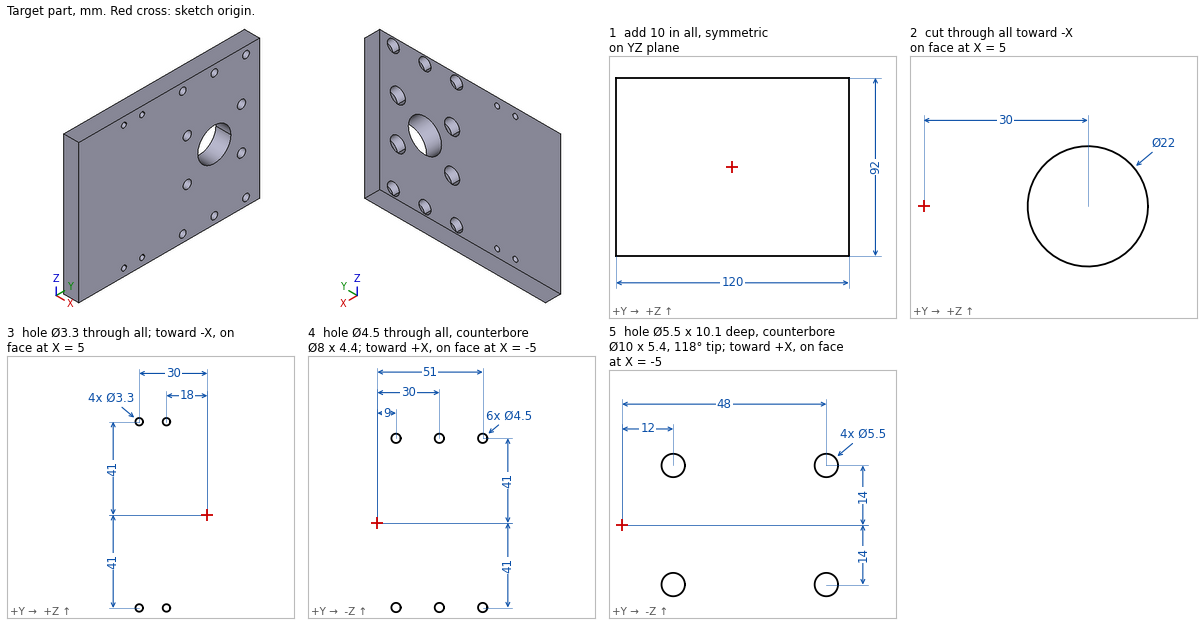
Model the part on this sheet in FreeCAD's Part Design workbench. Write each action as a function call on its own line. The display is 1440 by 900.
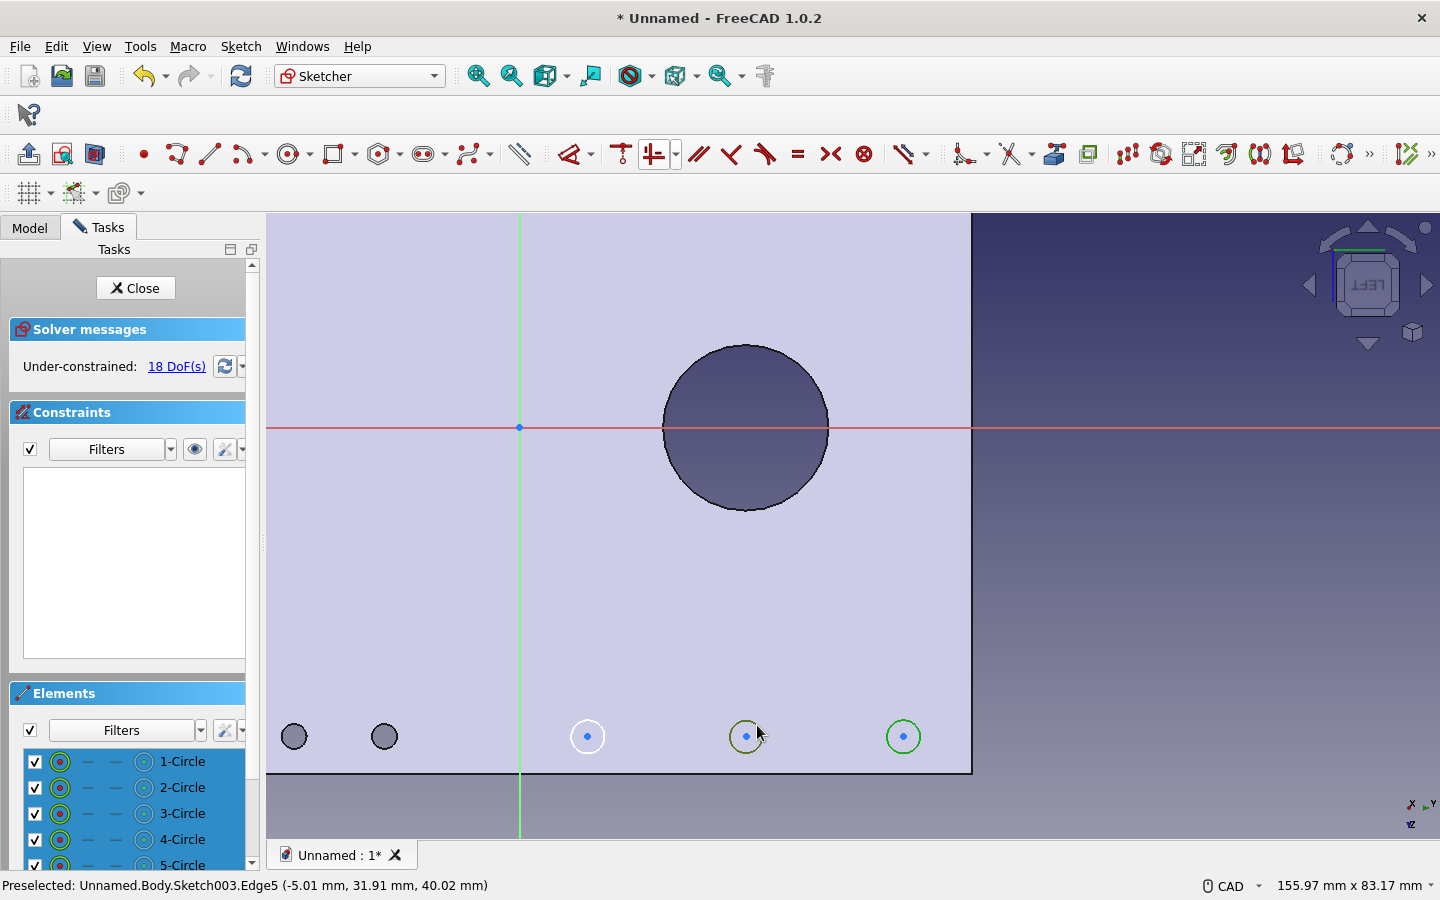
click(600, 725)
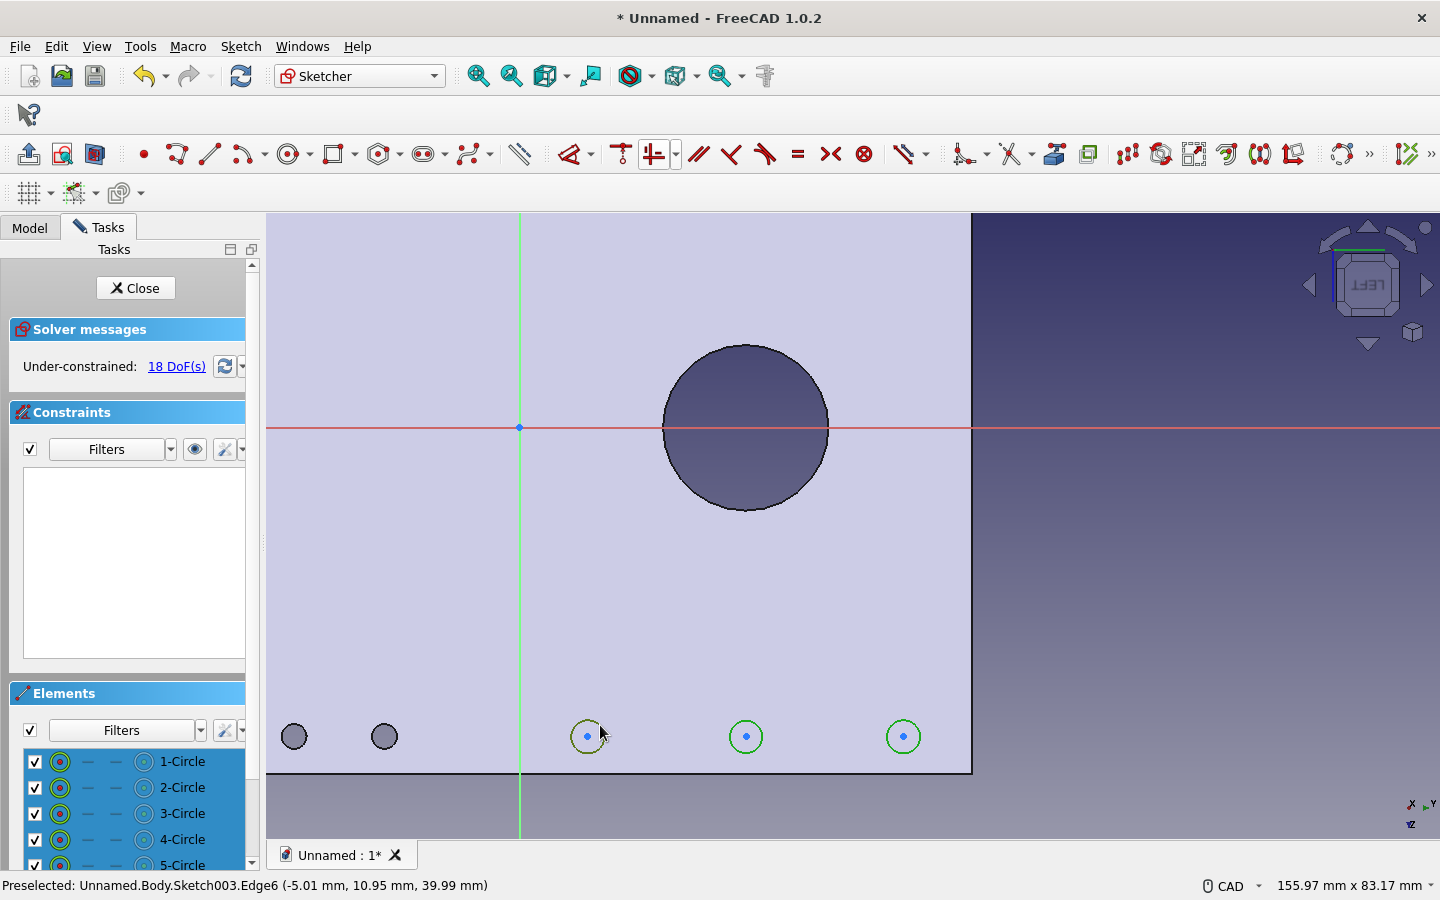
key(e)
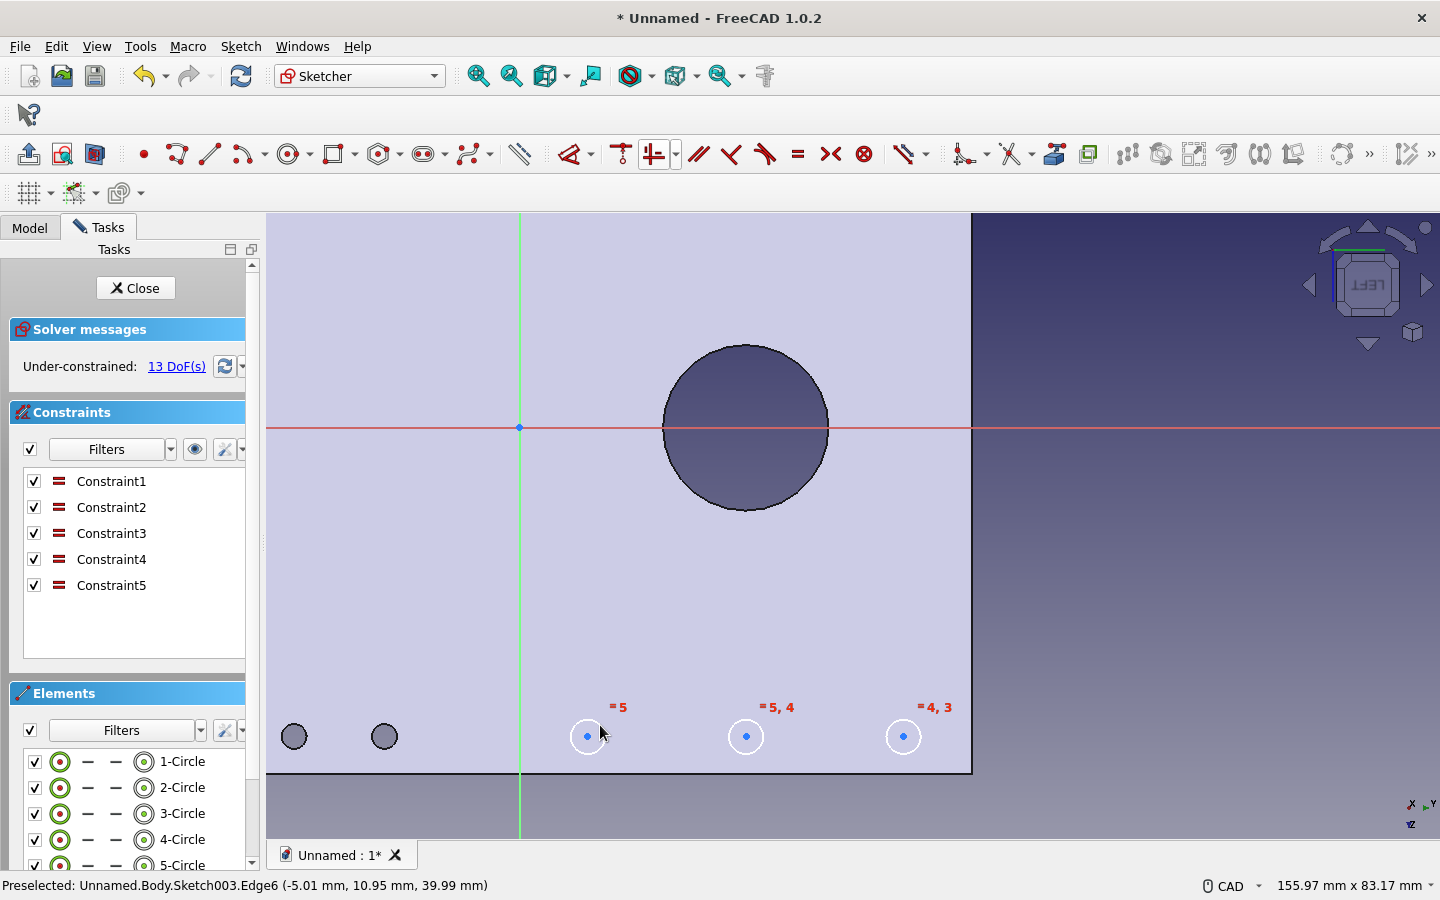
scroll(915, 726, down, 2)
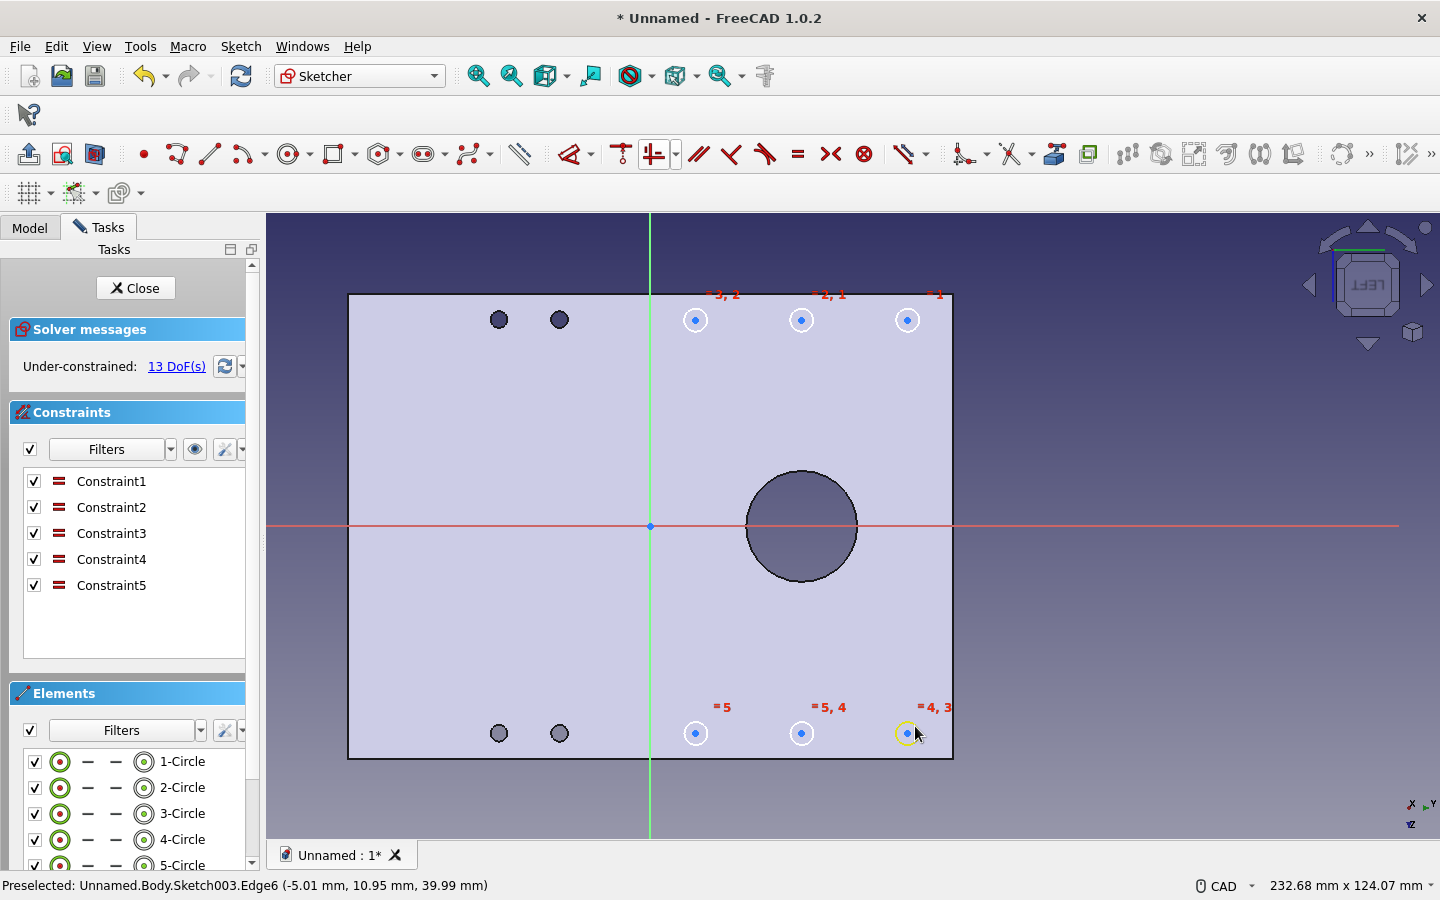
click(908, 320)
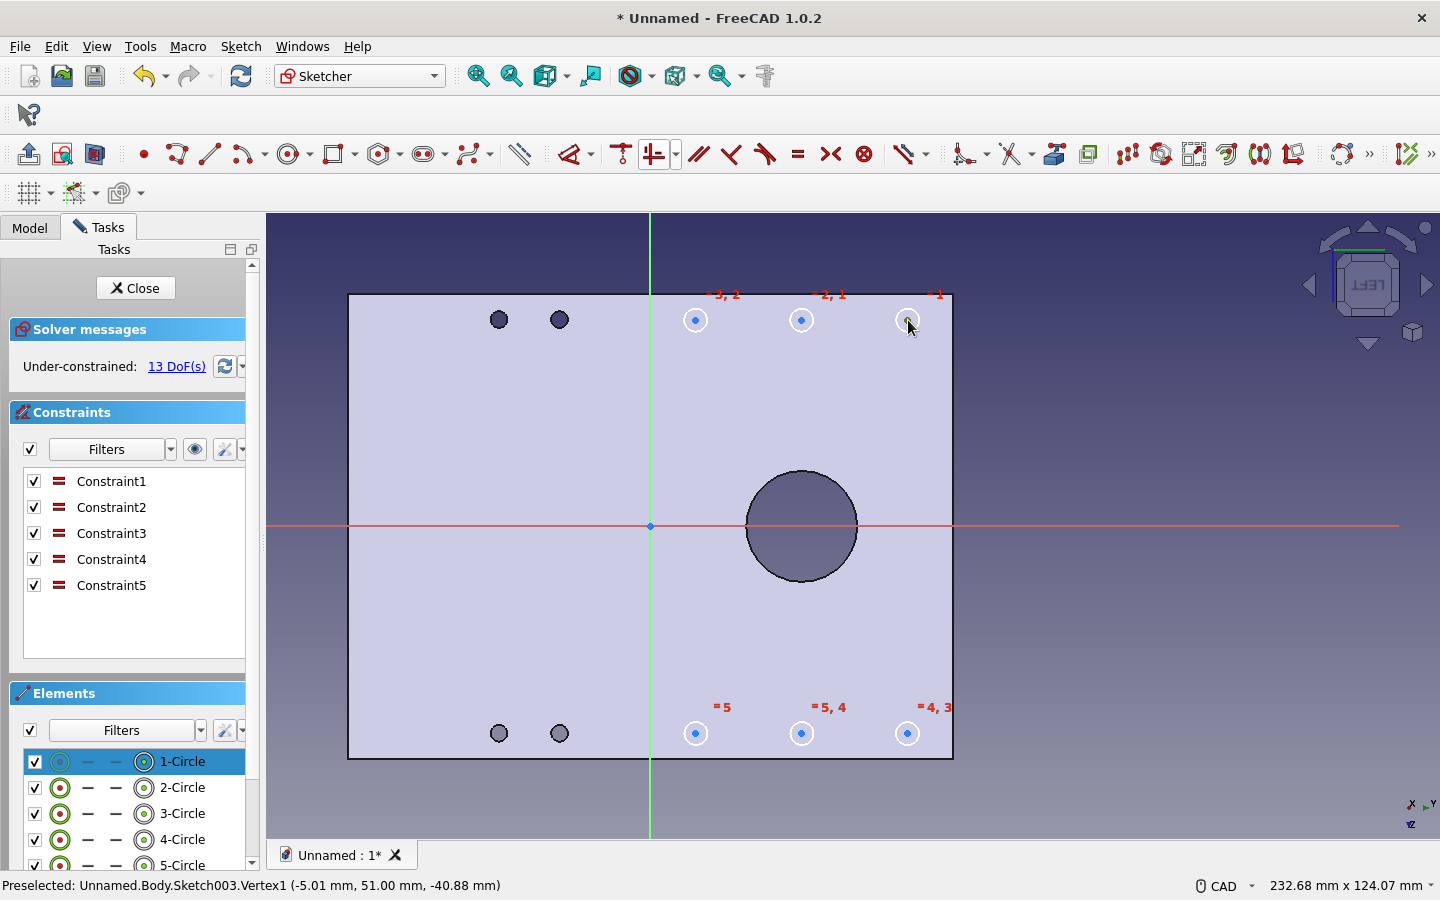
click(802, 320)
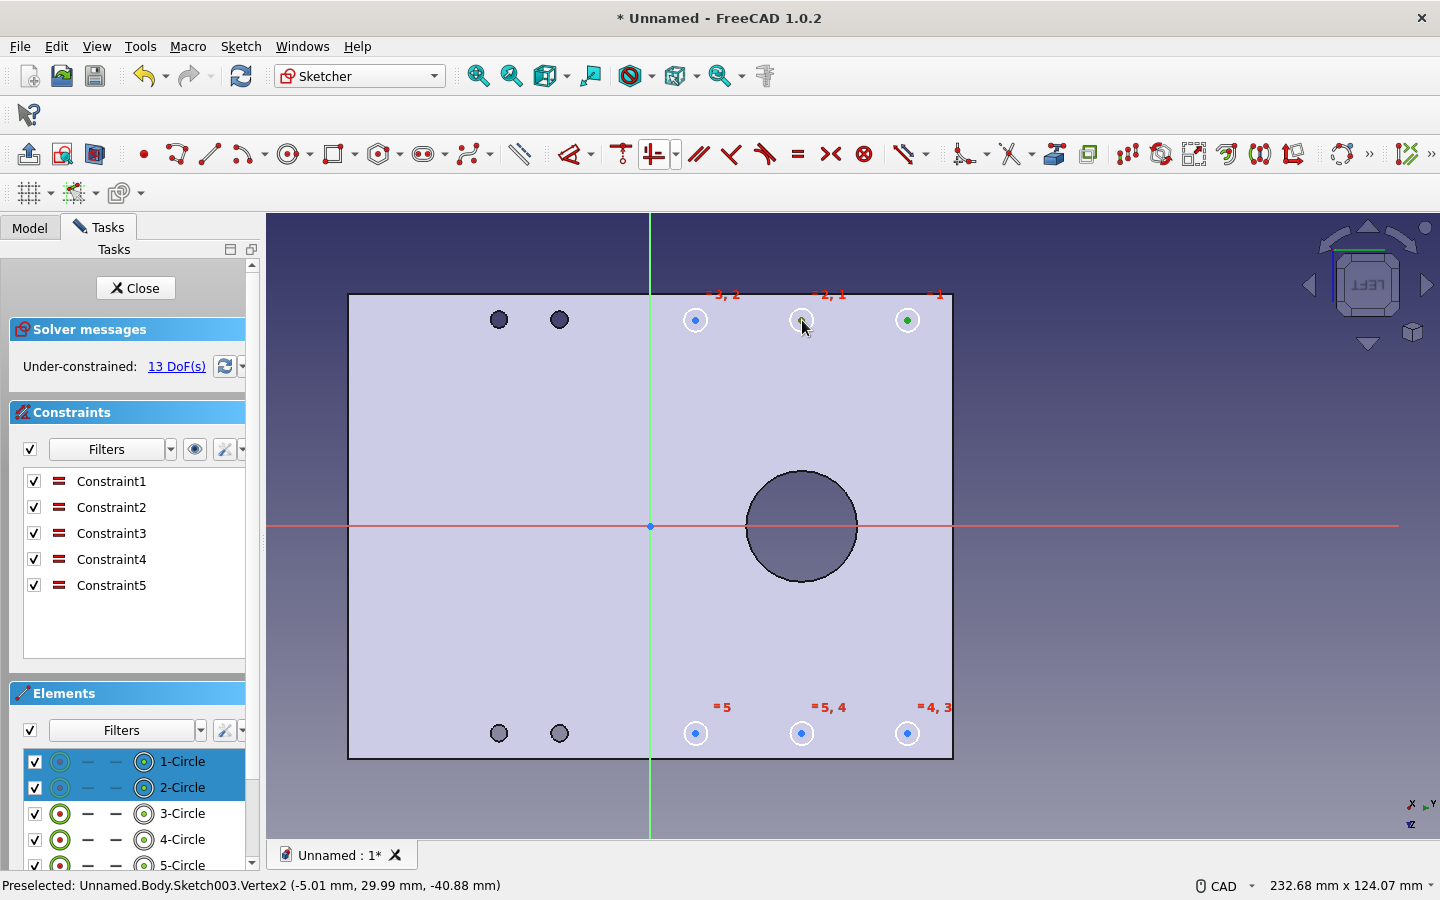
click(676, 154)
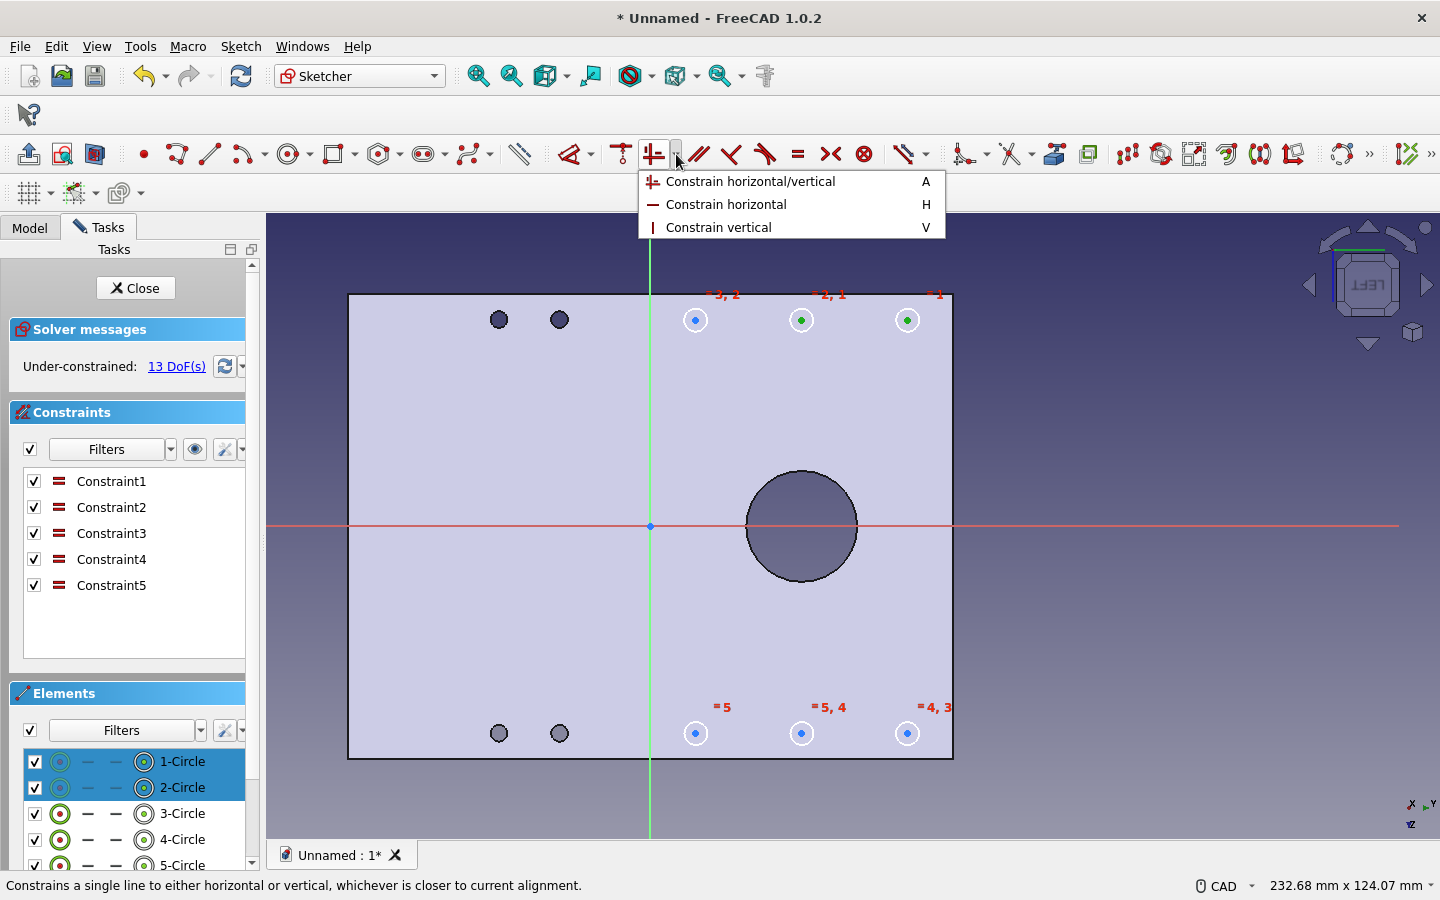
click(792, 204)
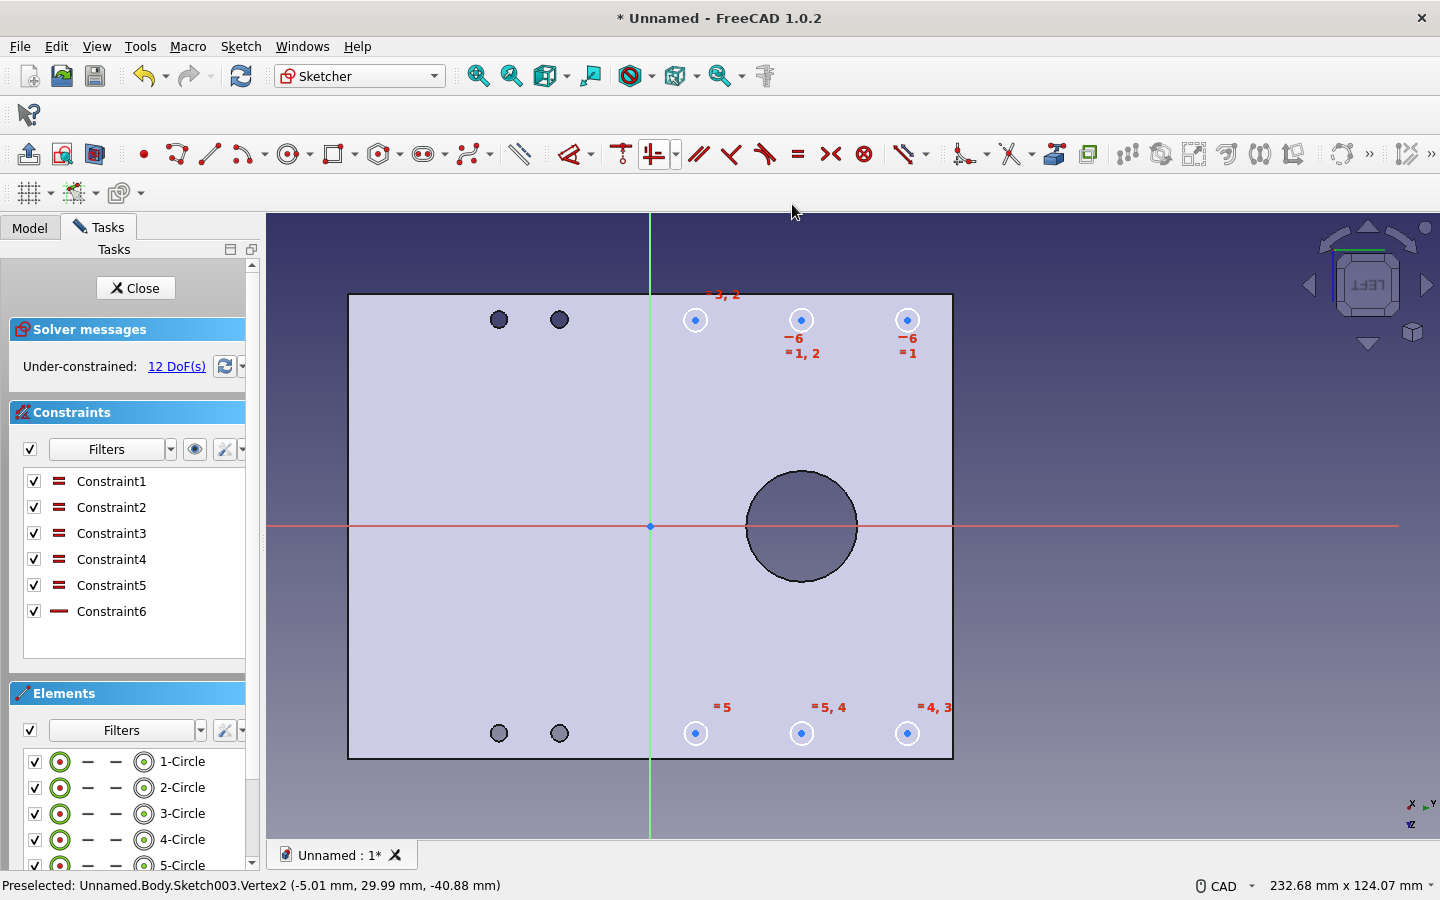
click(802, 320)